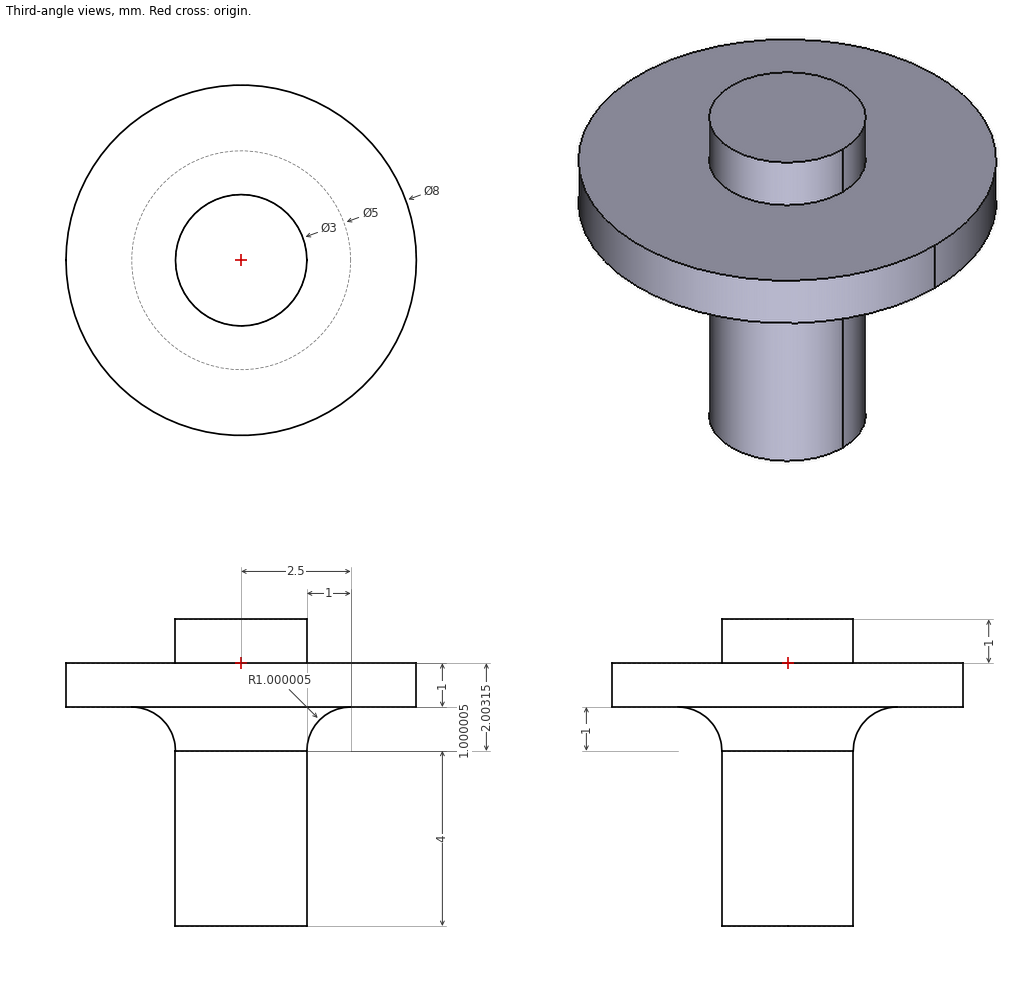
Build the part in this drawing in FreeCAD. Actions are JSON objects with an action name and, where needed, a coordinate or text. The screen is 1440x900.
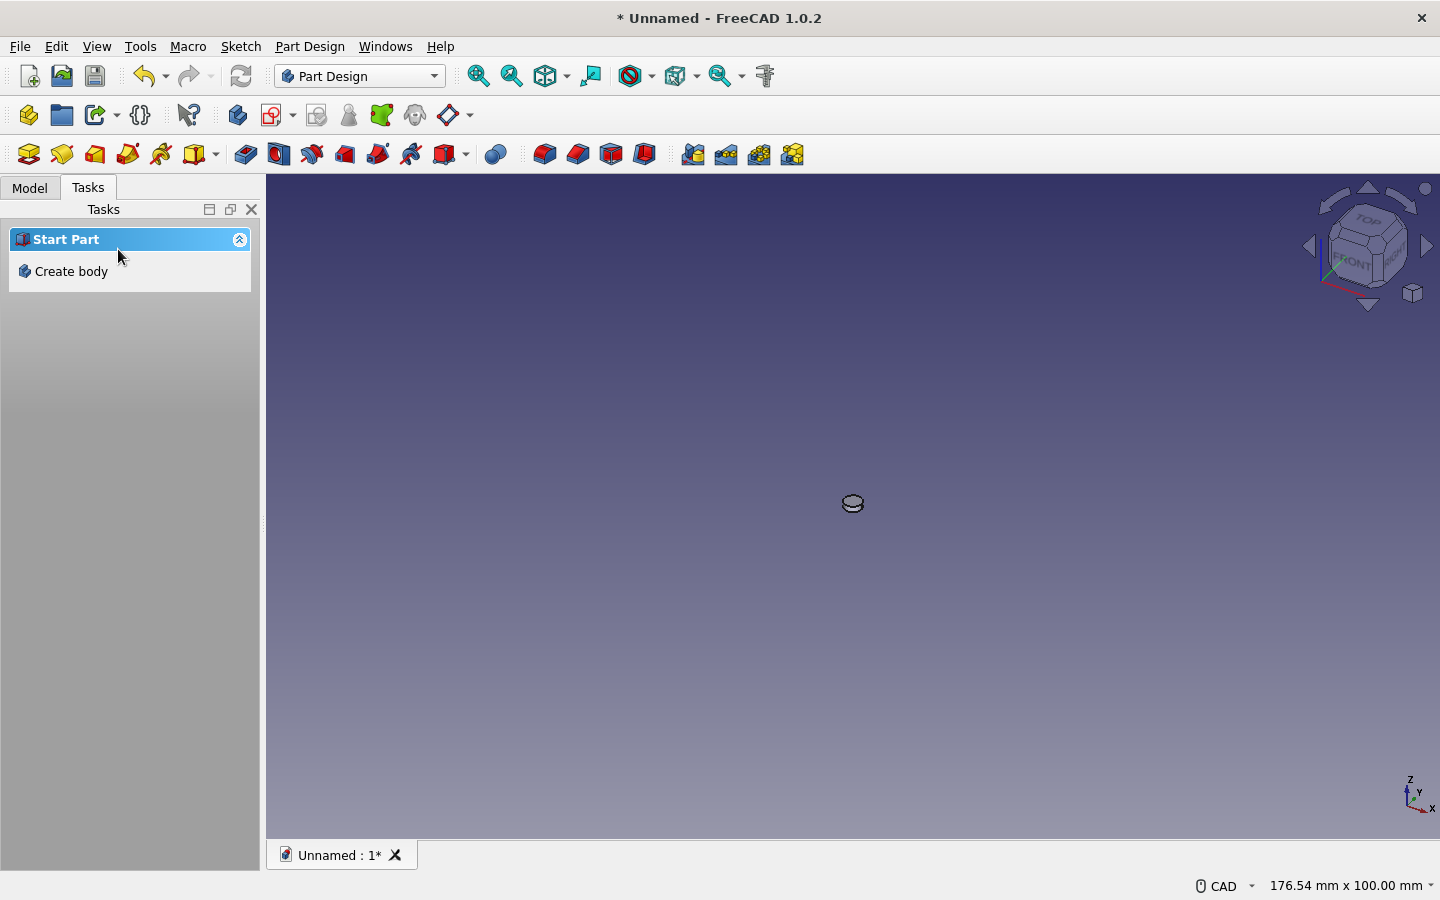
{"action": "left_click", "coordinate": [479, 76]}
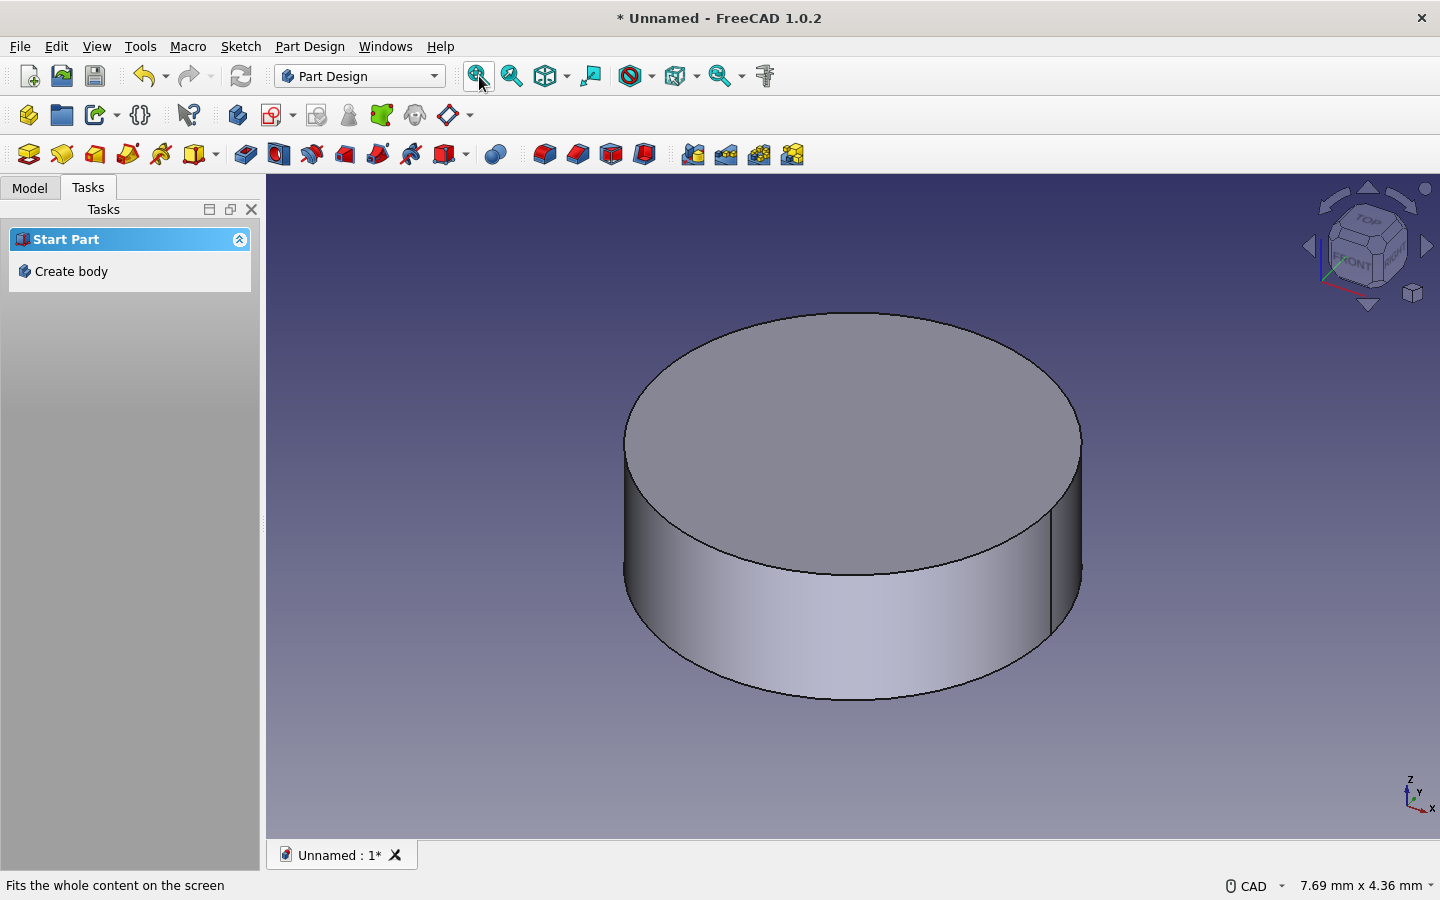
{"action": "key", "text": "5"}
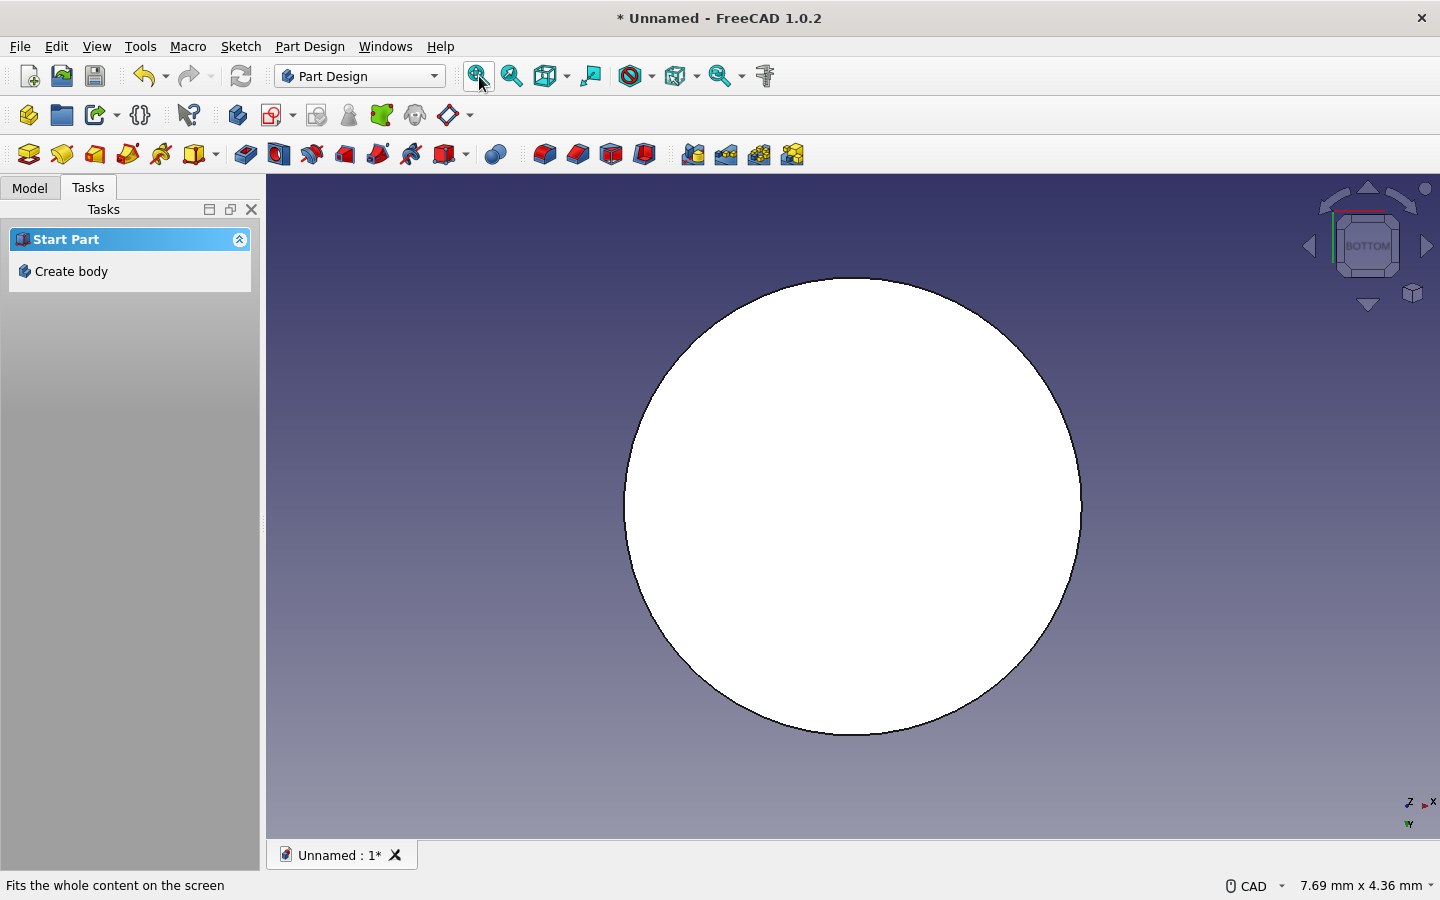
{"action": "left_click", "coordinate": [853, 505]}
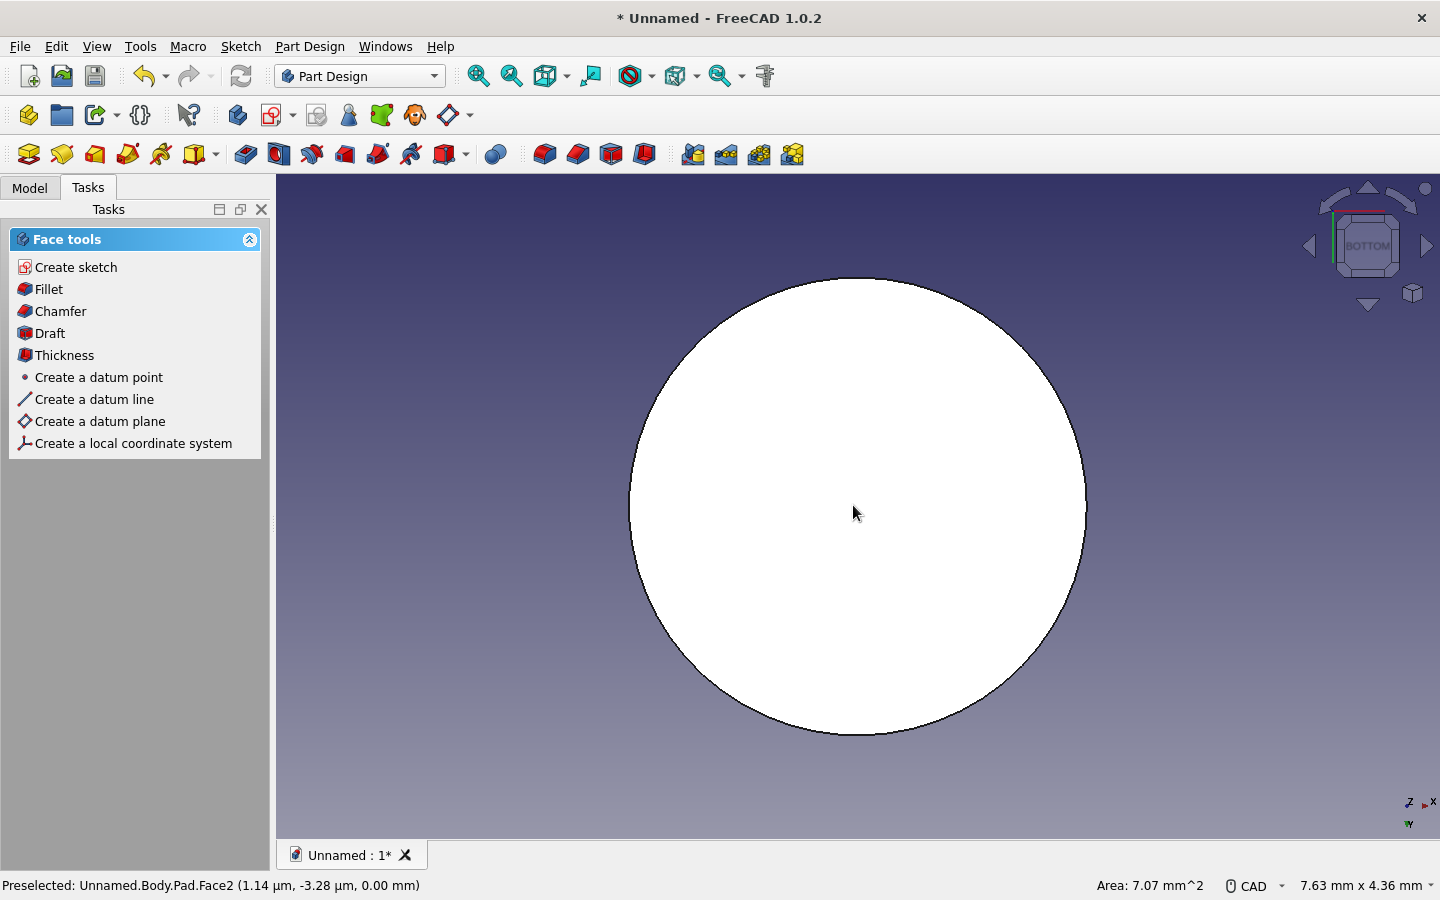
{"action": "left_click", "coordinate": [270, 116]}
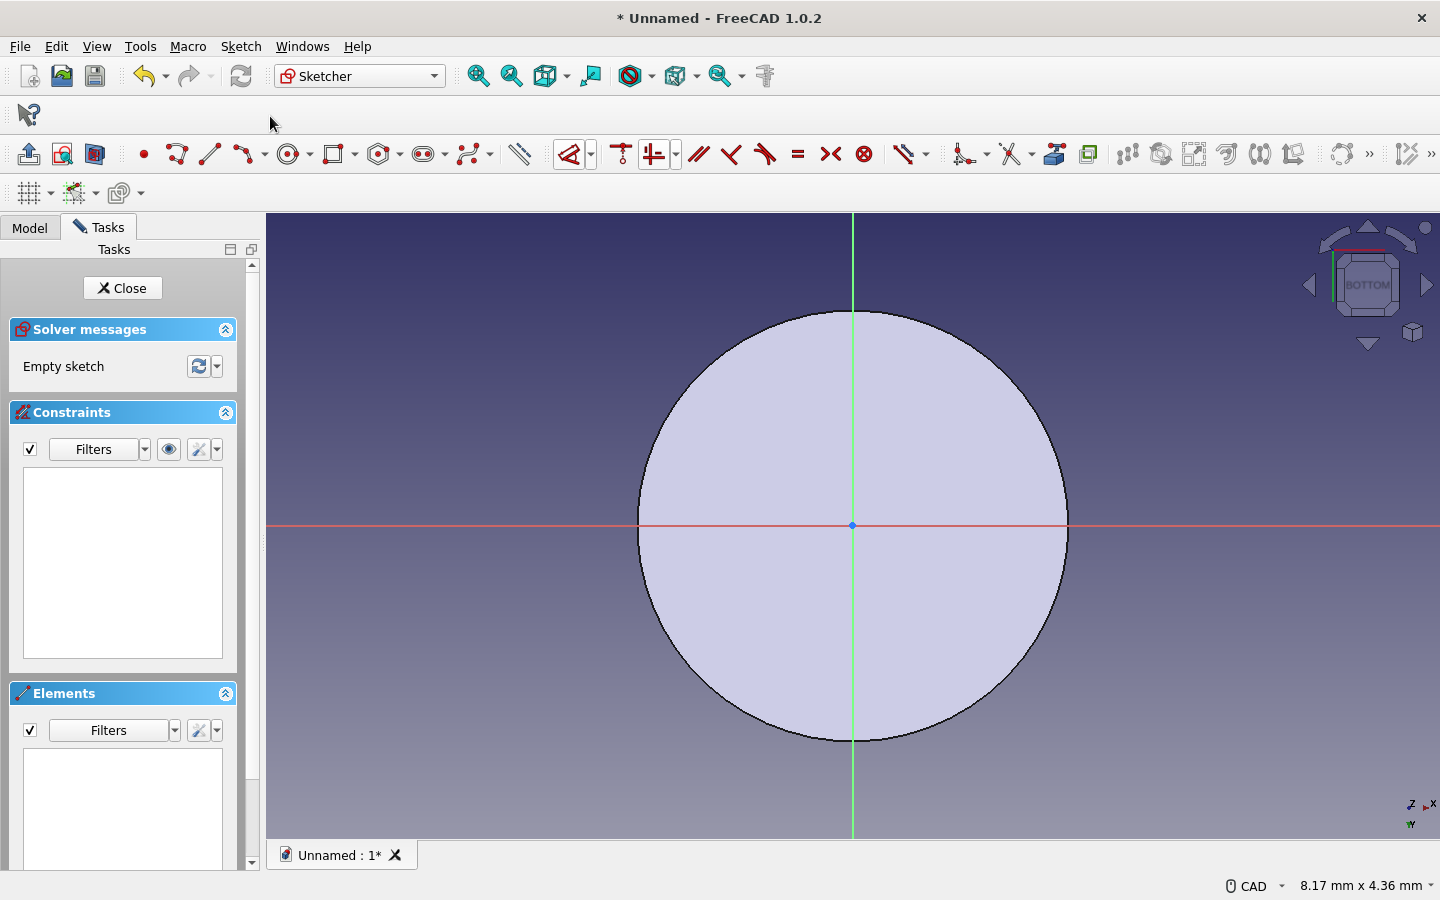
{"action": "scroll", "coordinate": [745, 526], "scroll_direction": "down", "scroll_amount": 5}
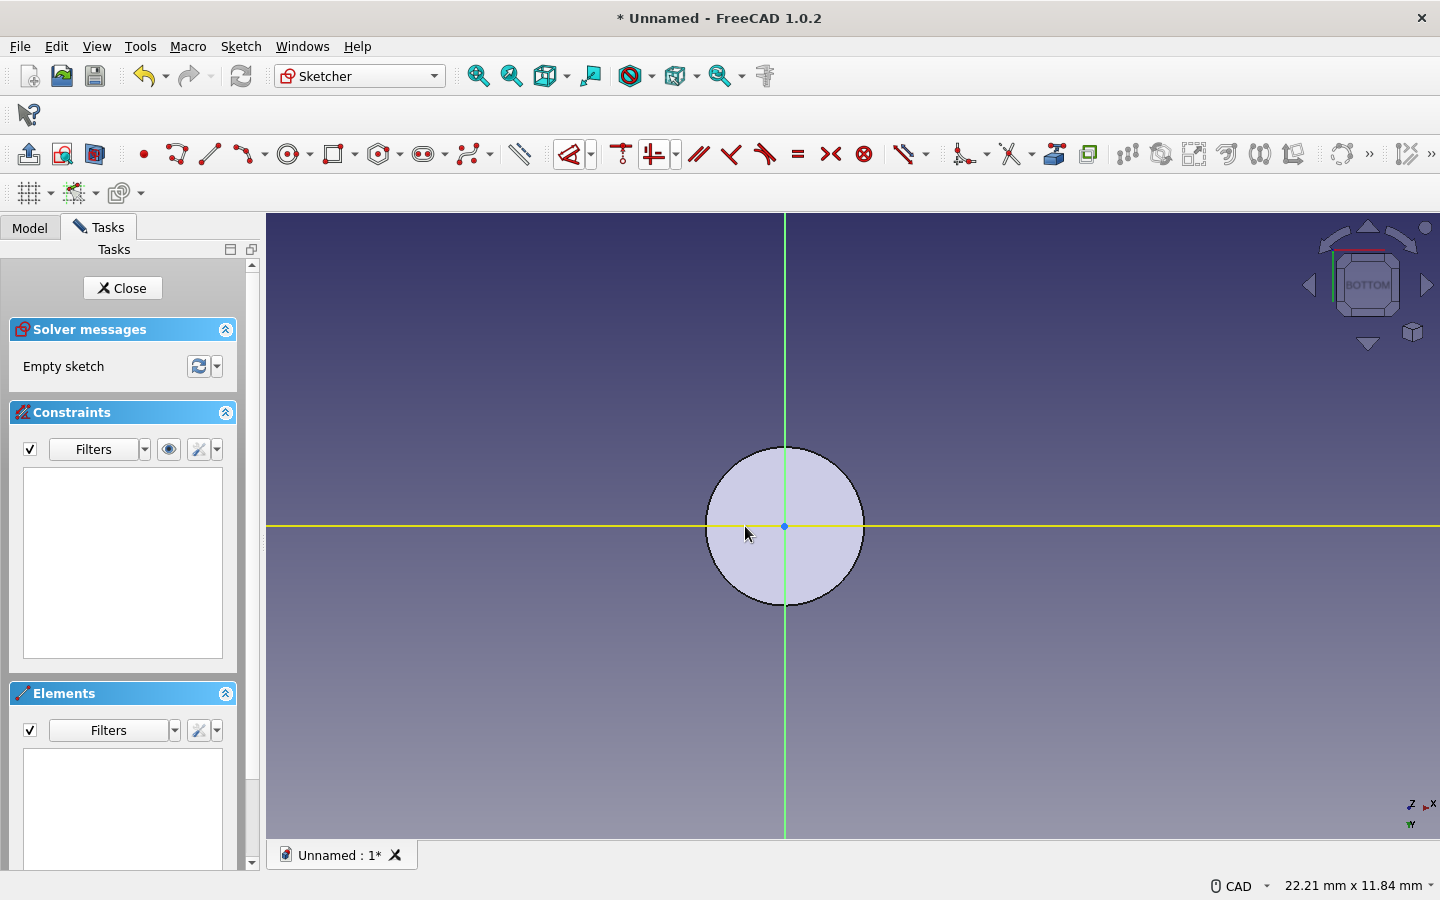
{"action": "left_click", "coordinate": [288, 154]}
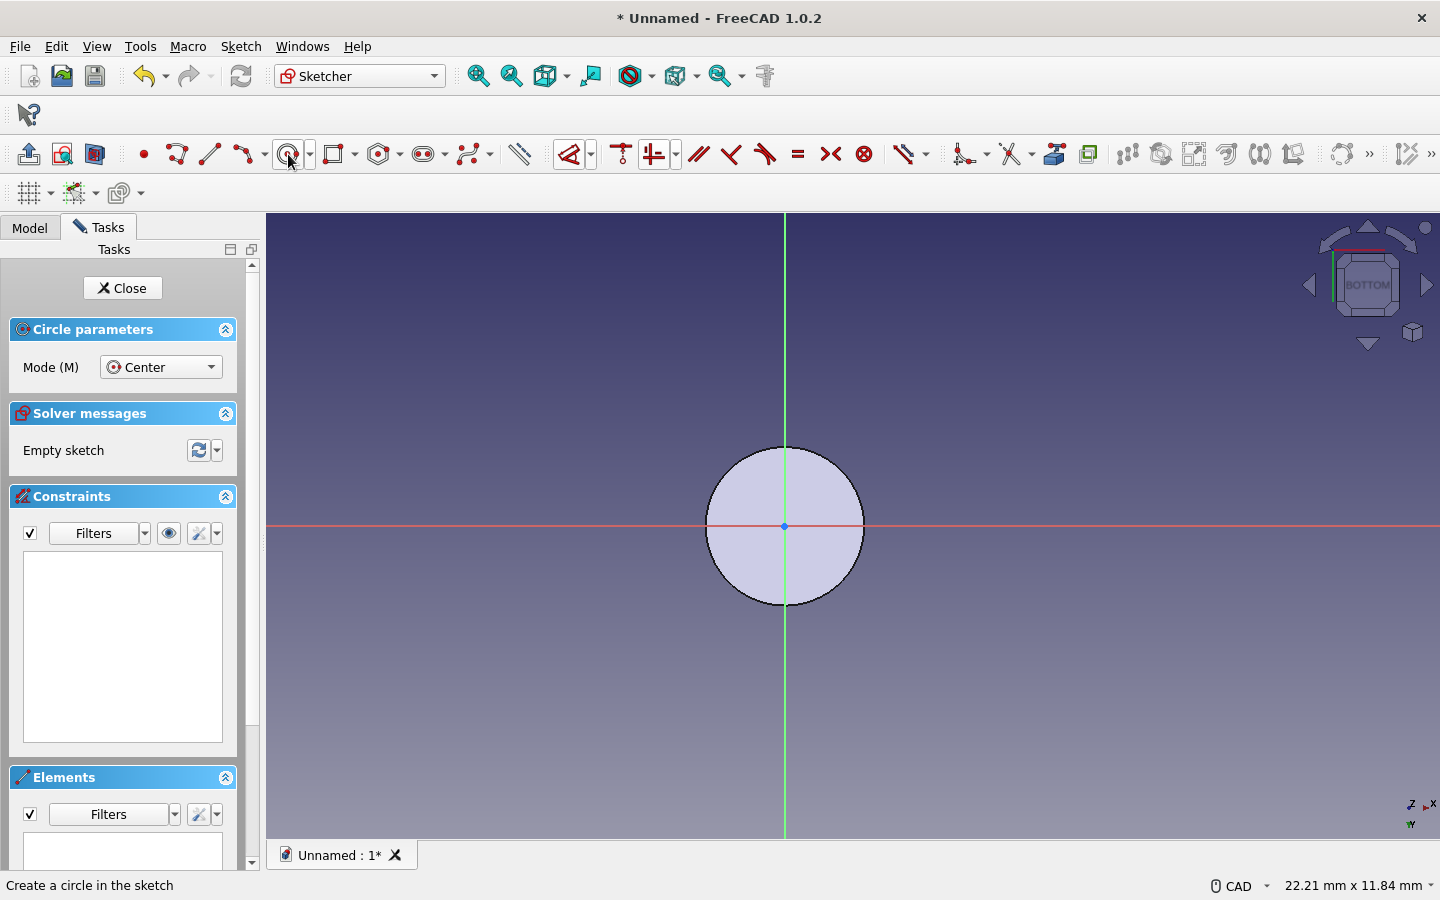
{"action": "left_click", "coordinate": [785, 526]}
{"action": "left_click", "coordinate": [934, 377]}
{"action": "key", "text": "Escape"}